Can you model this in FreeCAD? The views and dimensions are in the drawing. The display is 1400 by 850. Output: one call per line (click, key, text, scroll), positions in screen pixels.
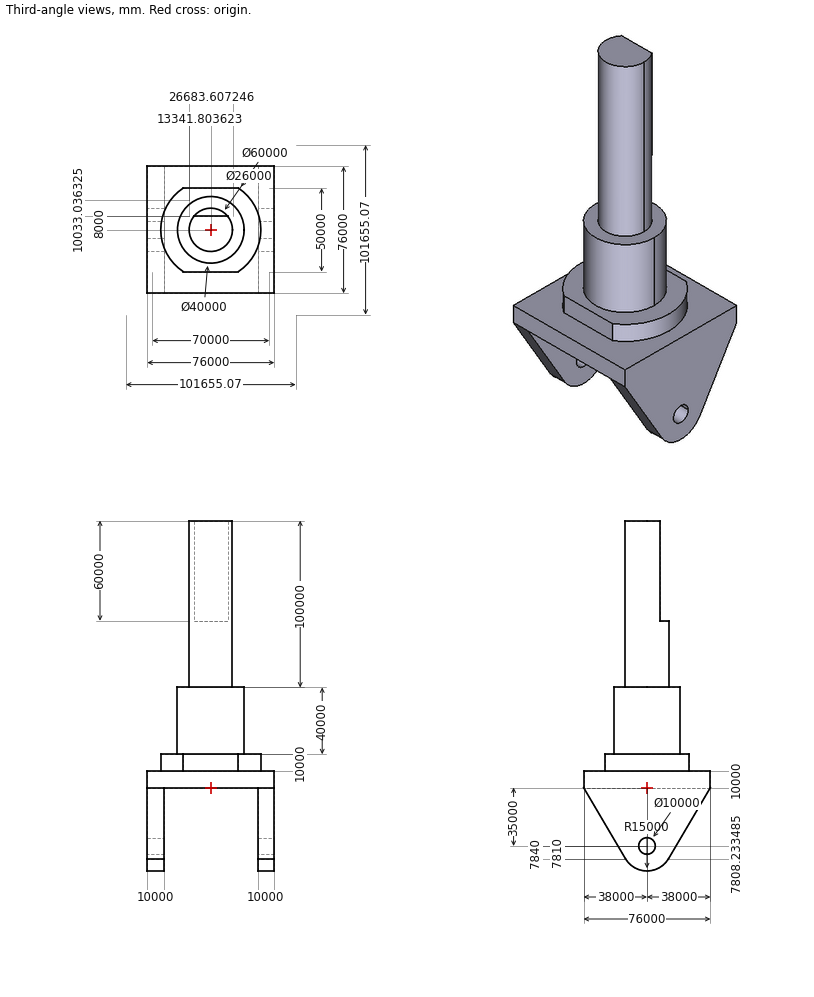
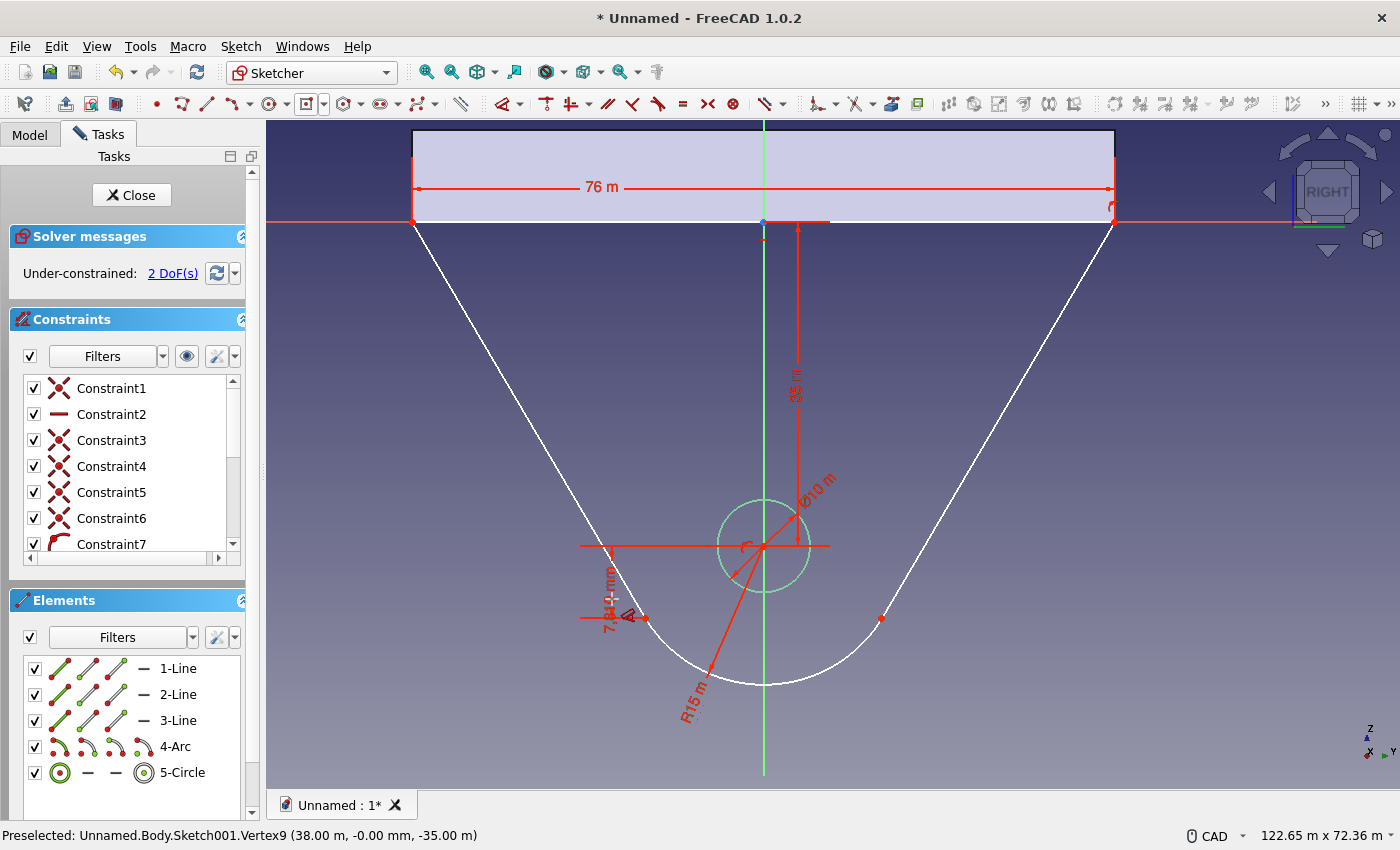
click(1115, 222)
click(939, 188)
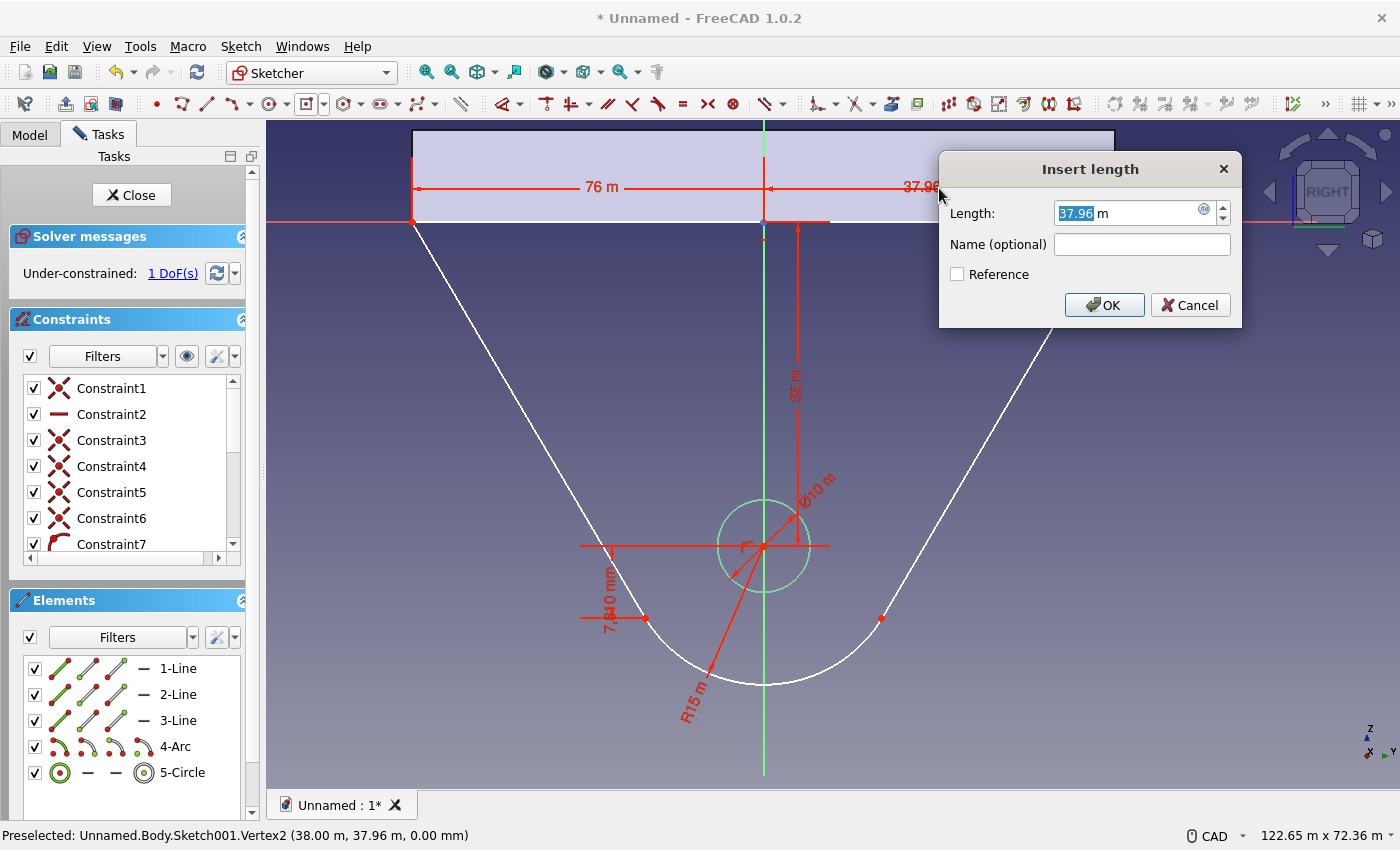
key(ctrl+a)
text(38000 mm)
key(Return)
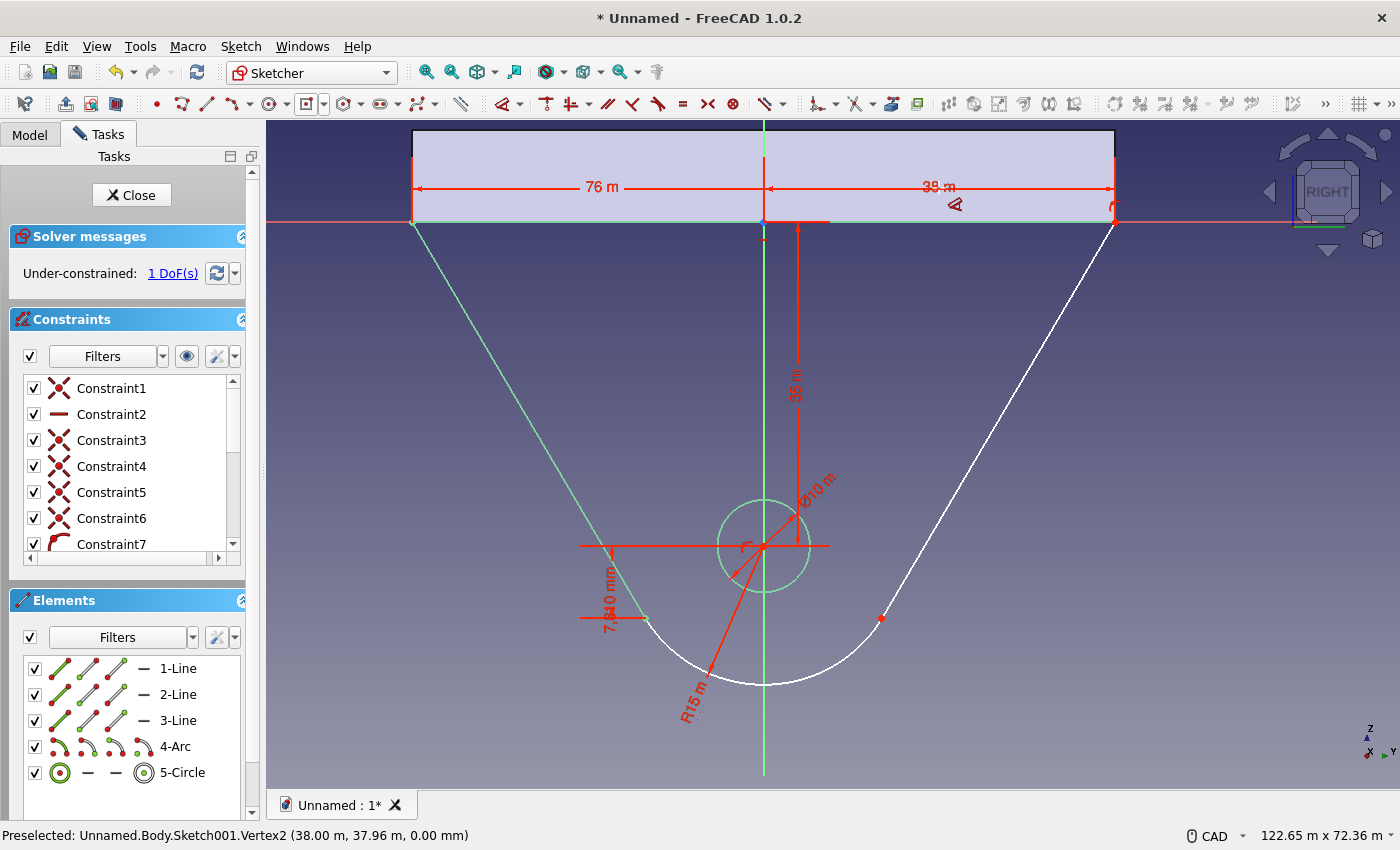
click(882, 619)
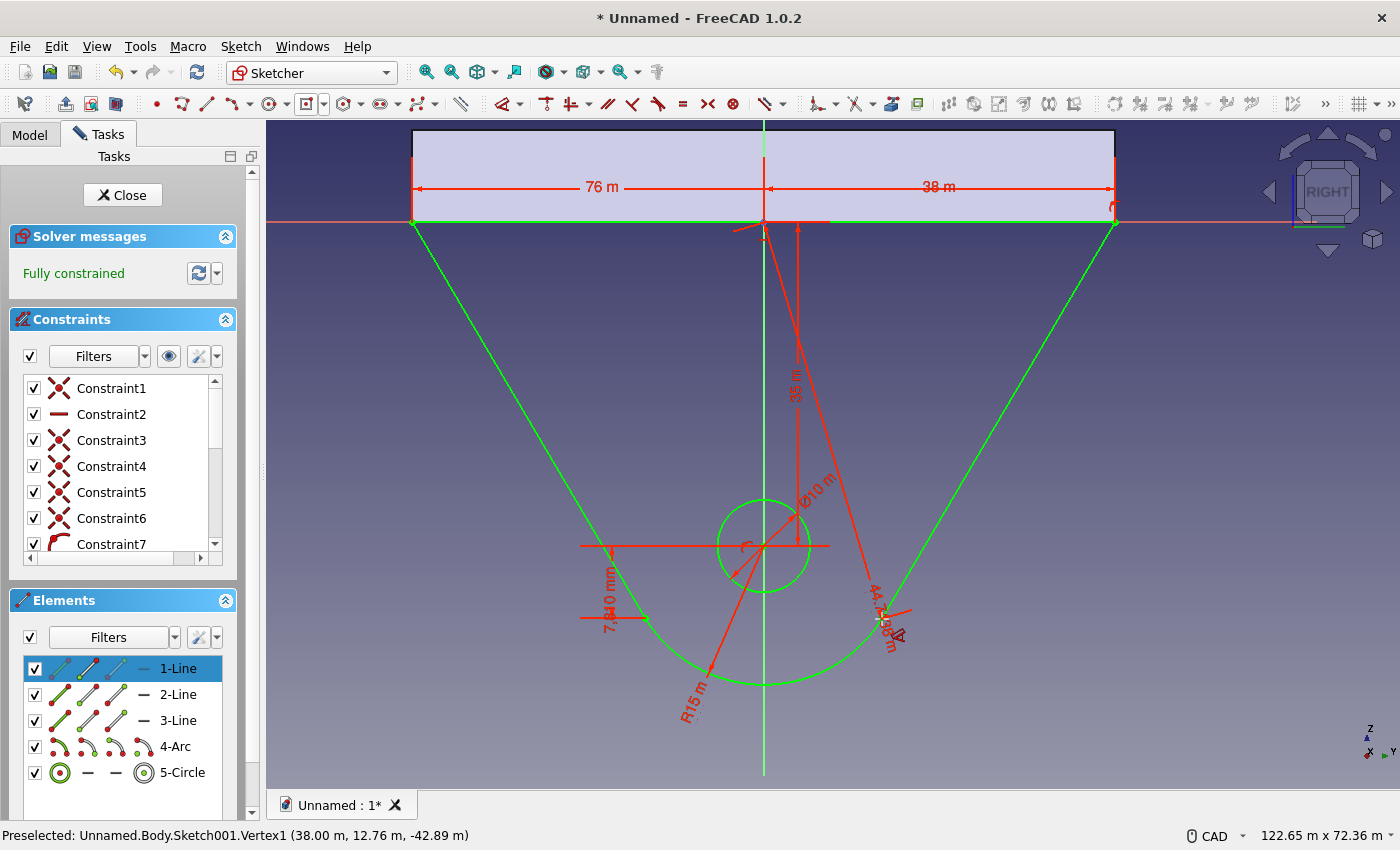
click(764, 546)
click(916, 599)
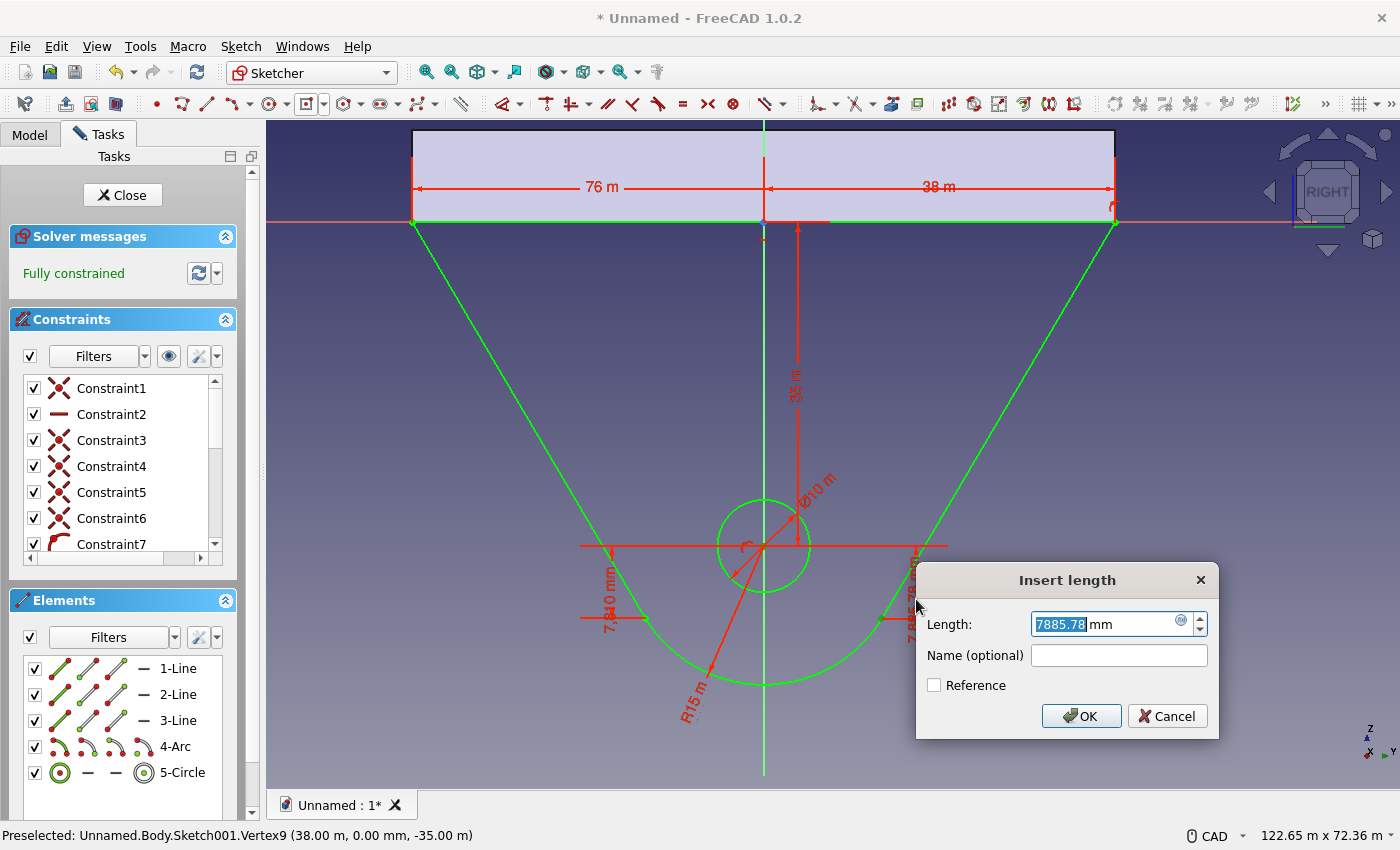
text(7808.233485)
key(Return)
key(Escape)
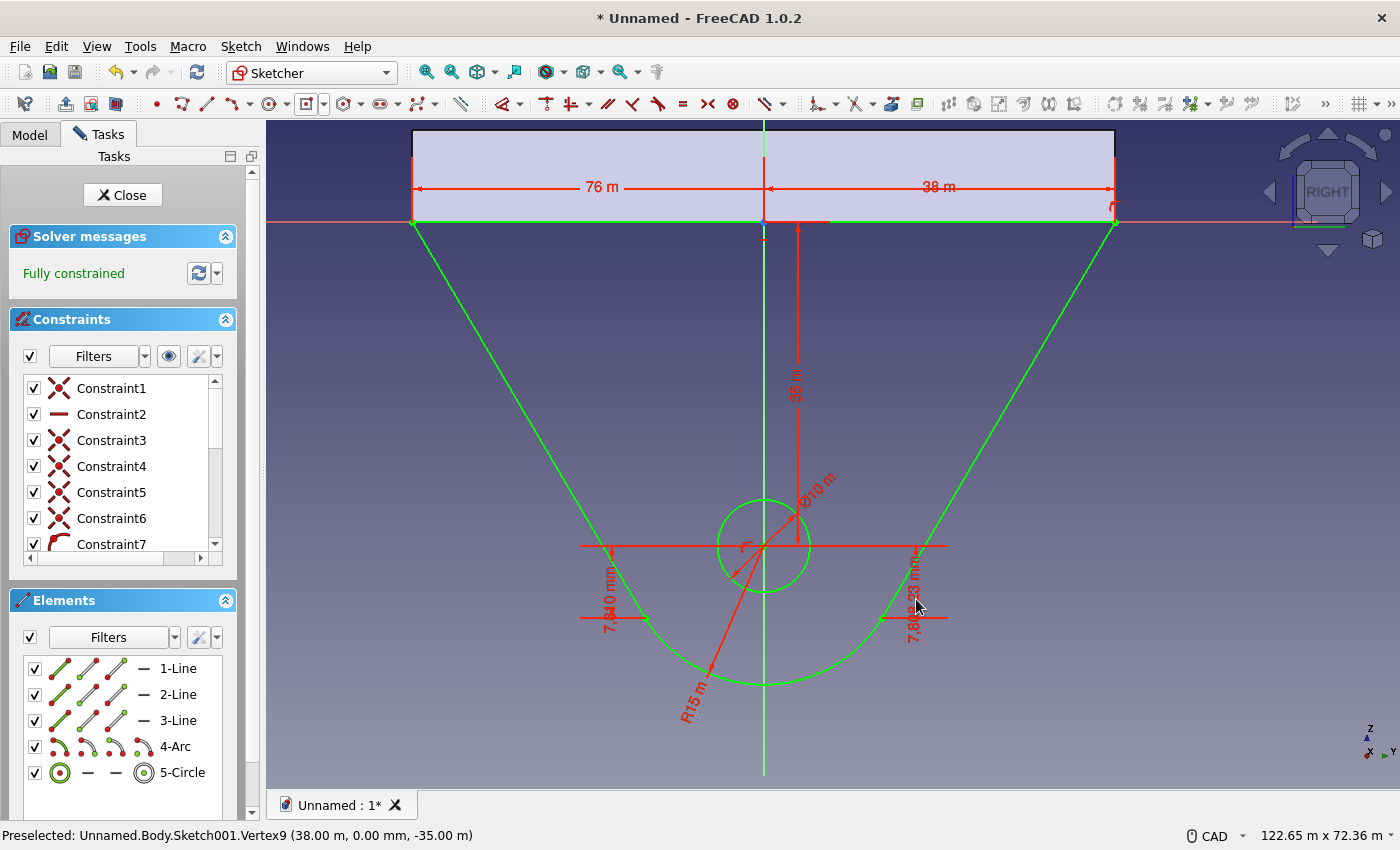
click(123, 195)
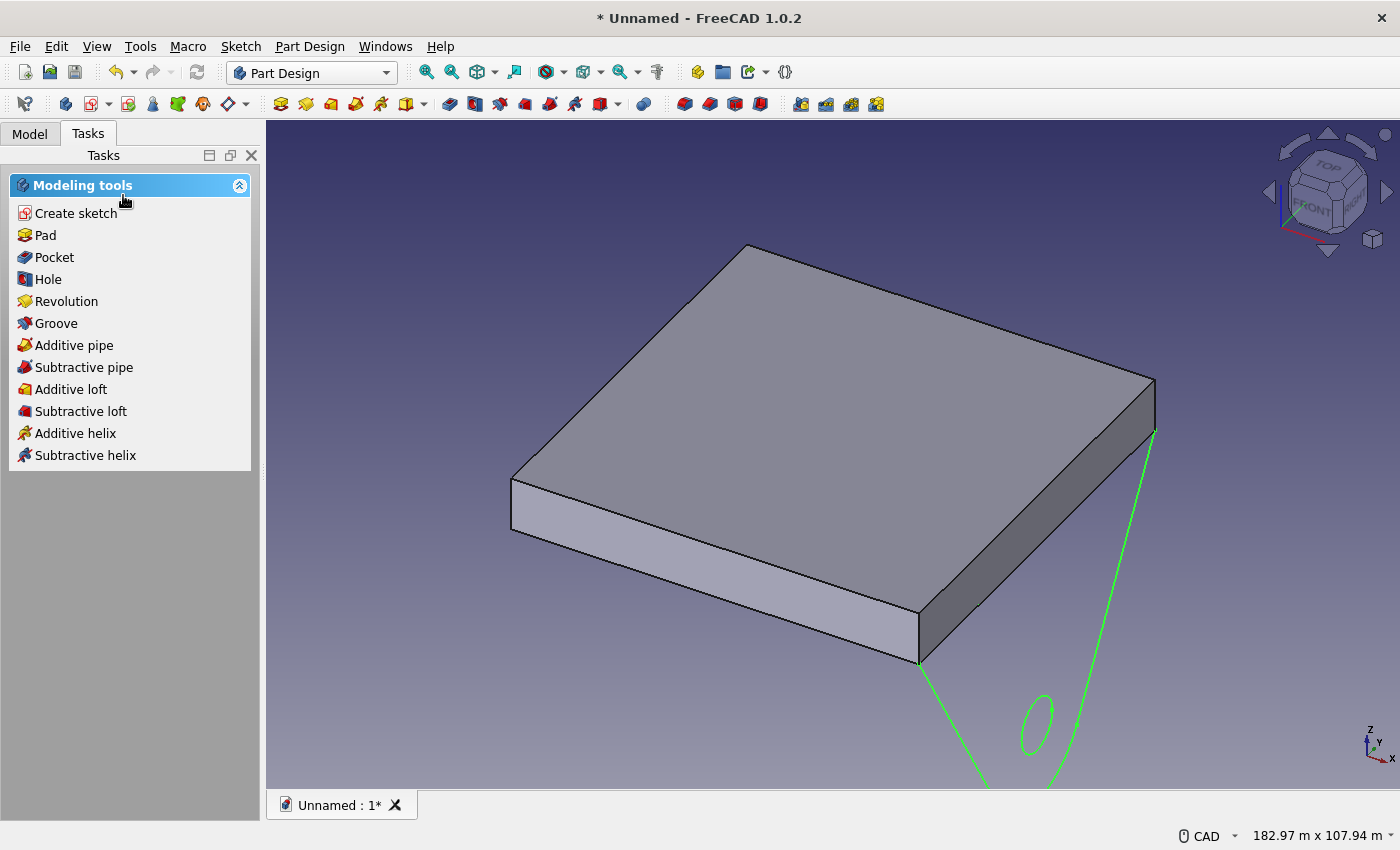
click(281, 104)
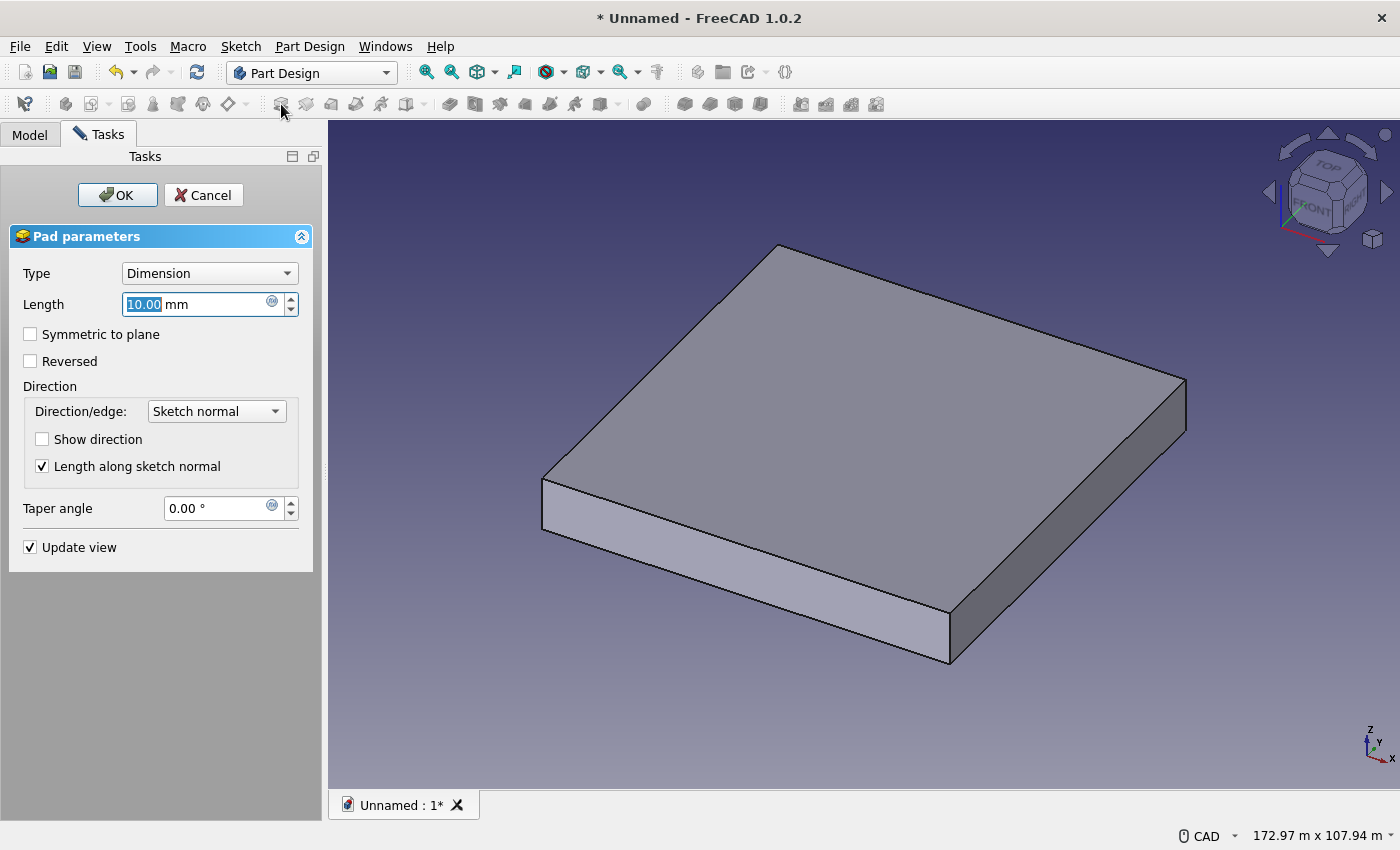
text(10000)
key(Tab)